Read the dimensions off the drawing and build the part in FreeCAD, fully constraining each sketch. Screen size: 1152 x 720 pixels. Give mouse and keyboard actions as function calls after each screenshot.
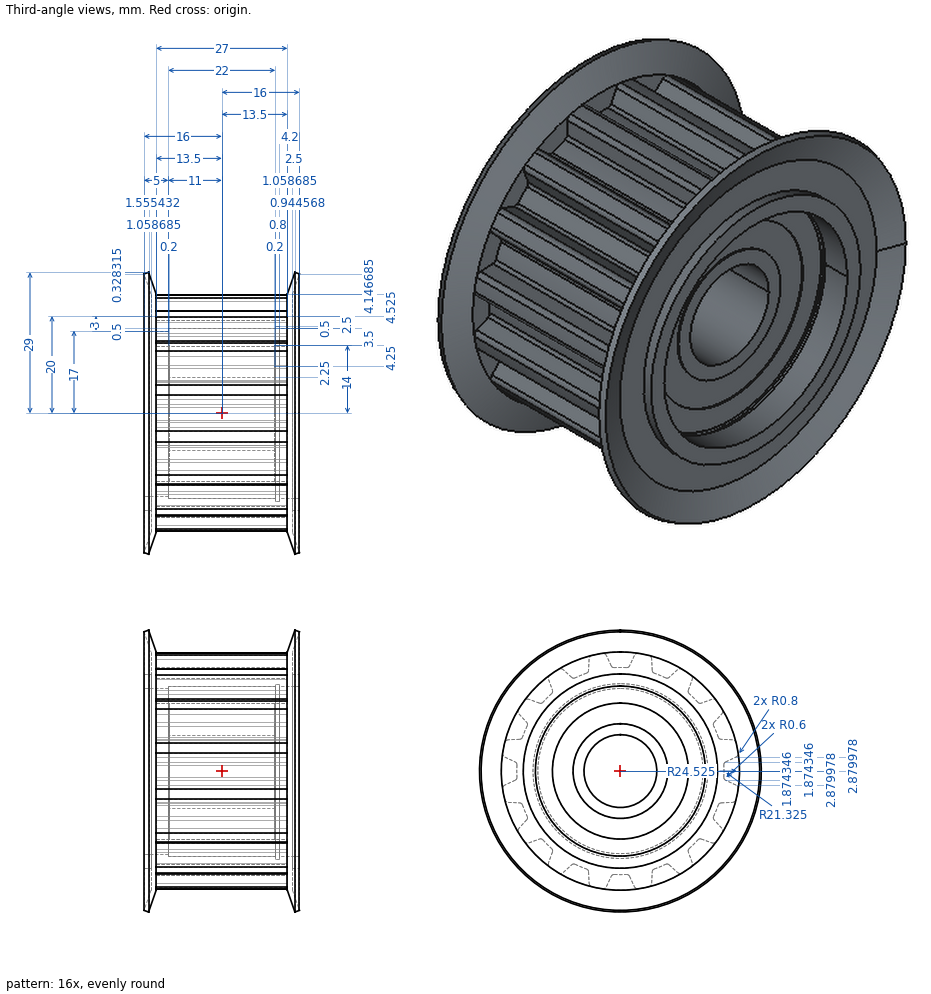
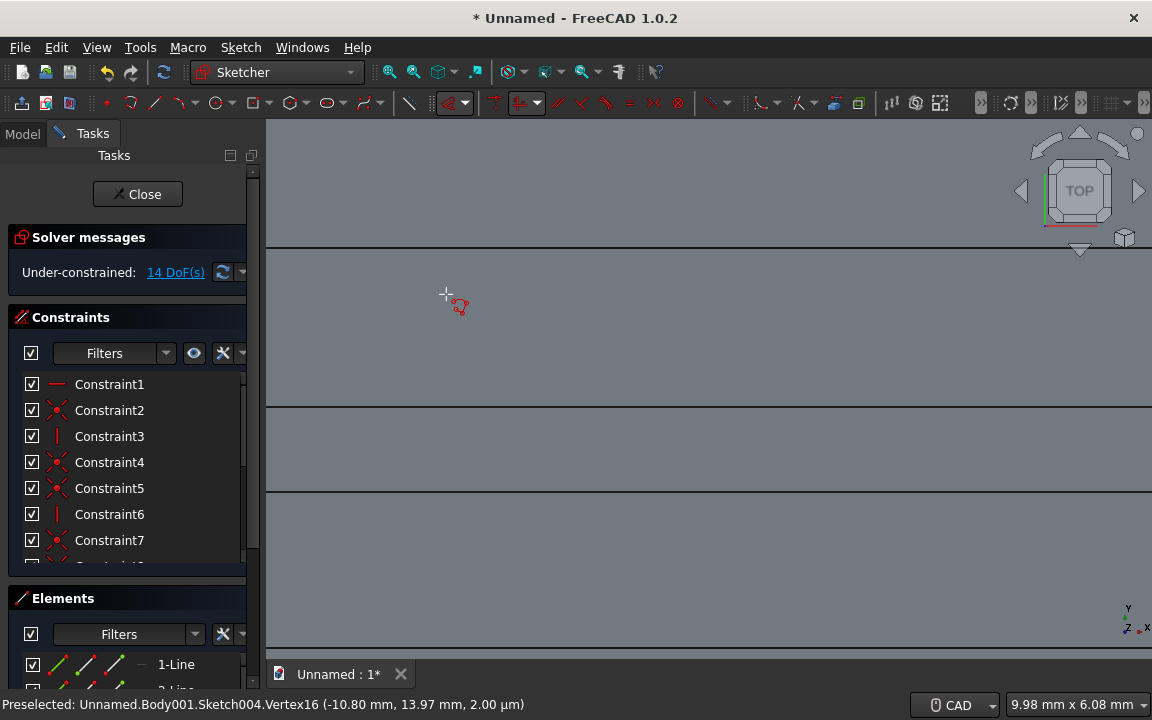
scroll(447, 295, down, 8)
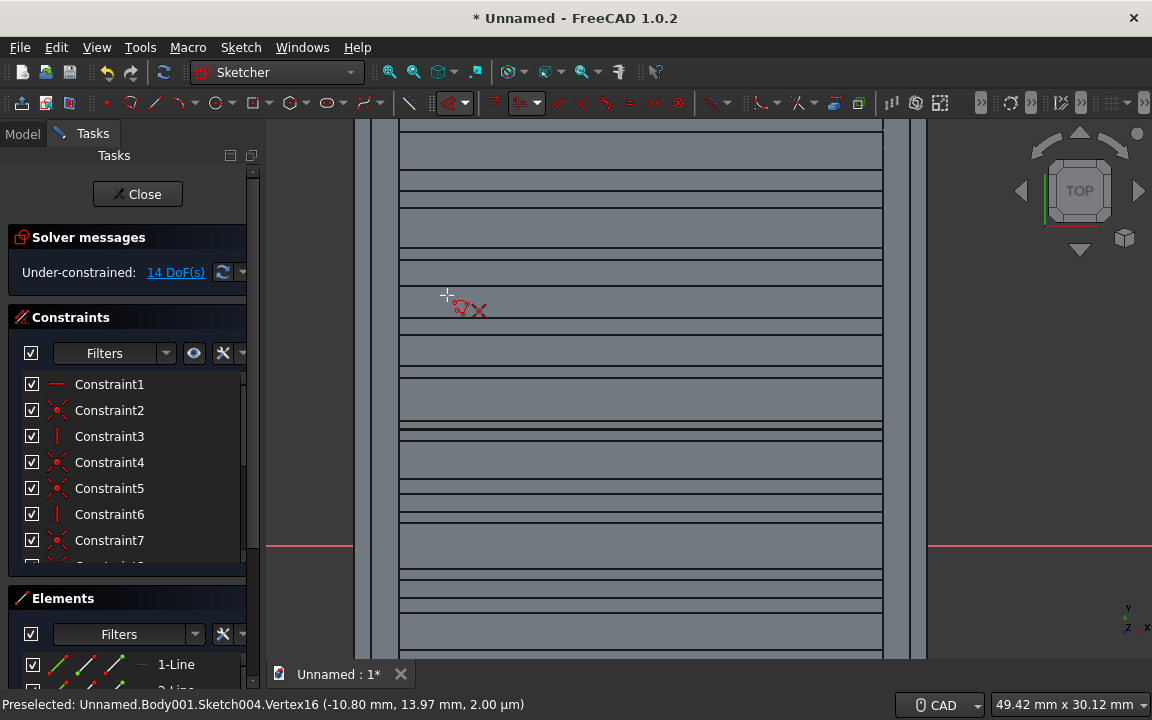
click(447, 371)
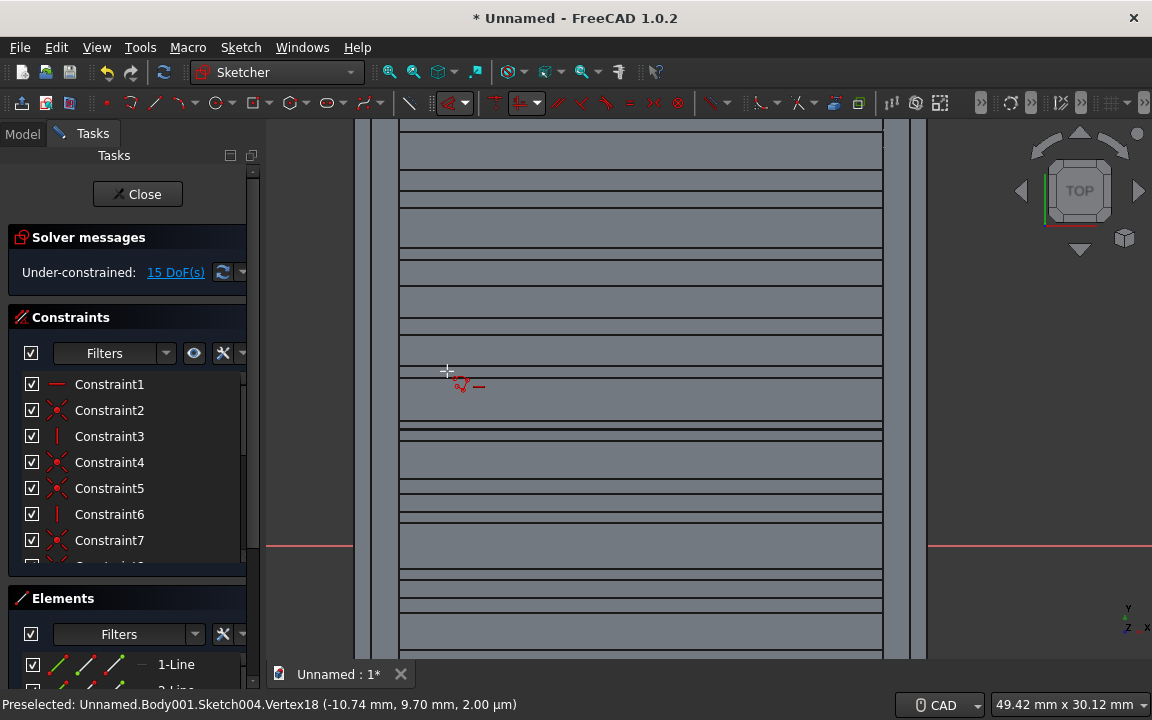
scroll(443, 371, up, 8)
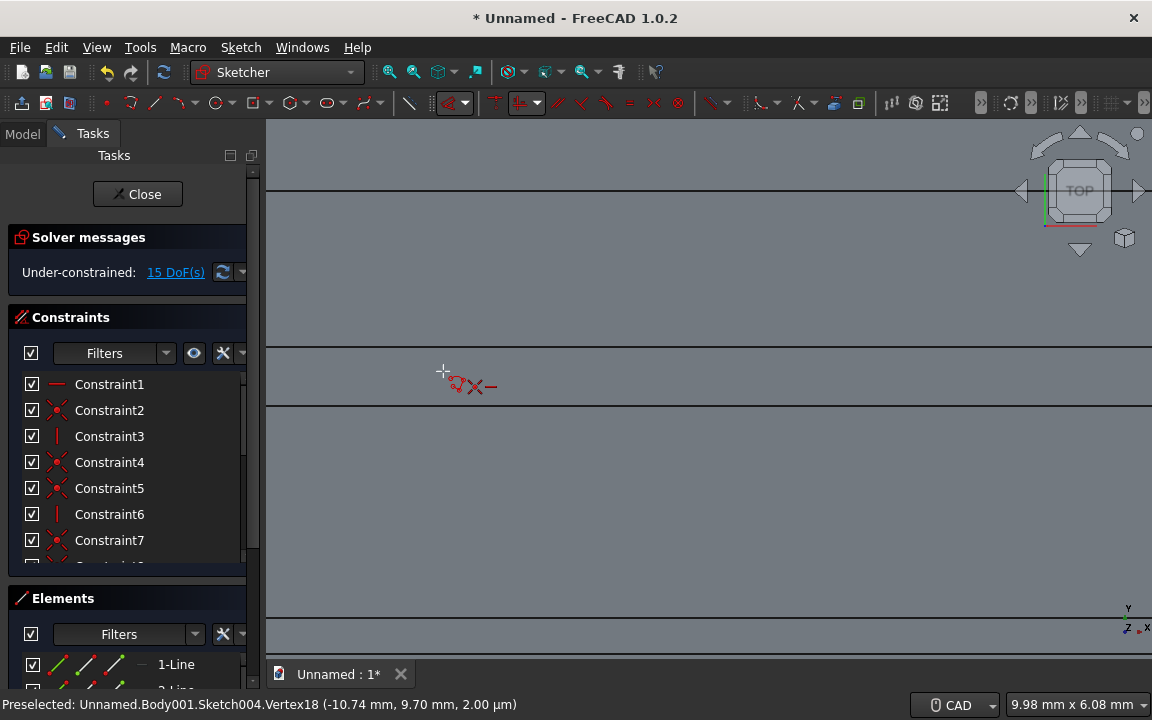
click(444, 369)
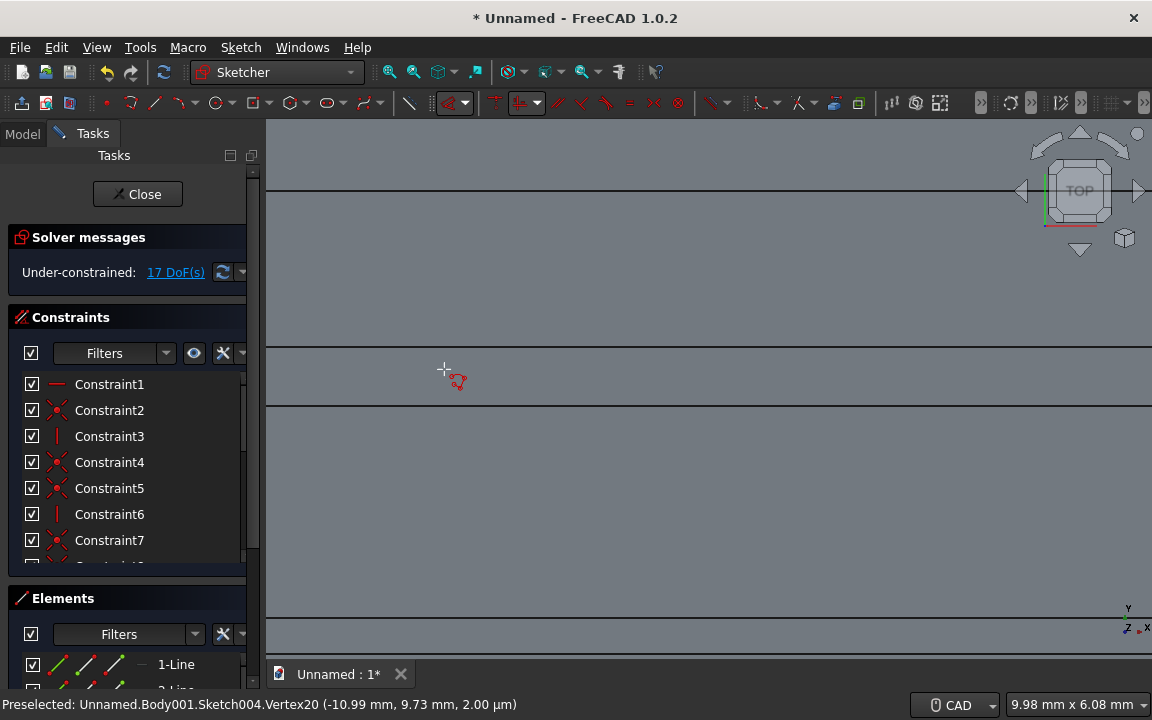
scroll(443, 371, down, 8)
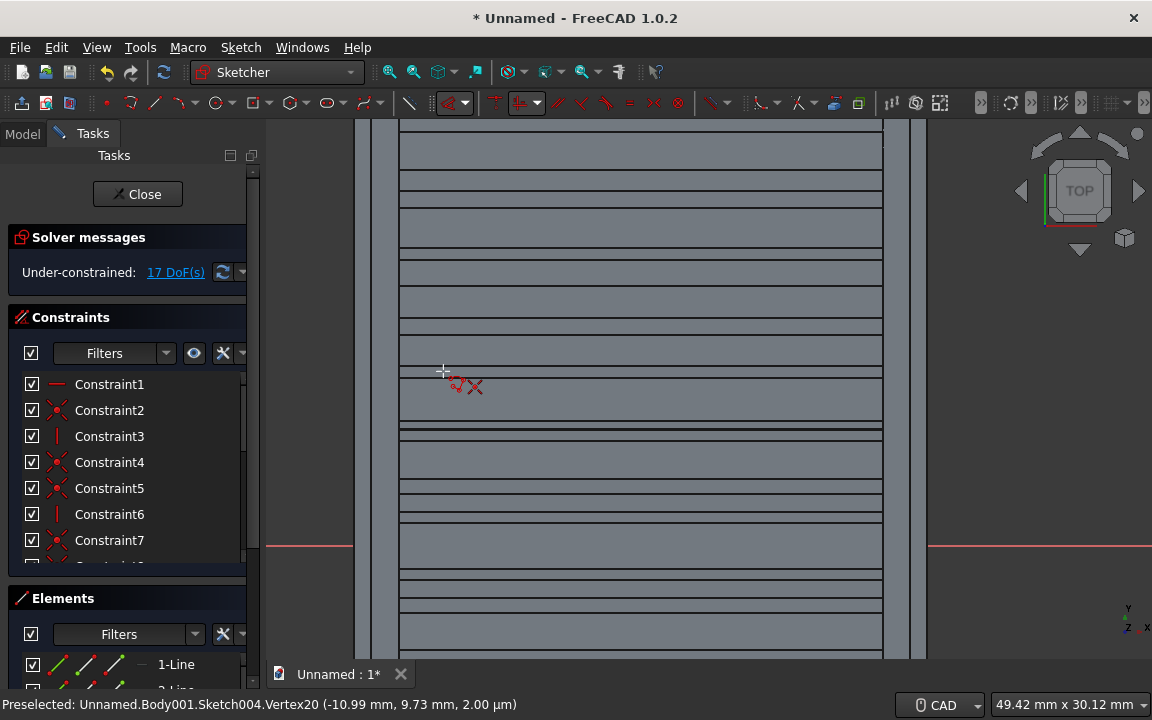
click(443, 412)
key(Escape)
key(Escape)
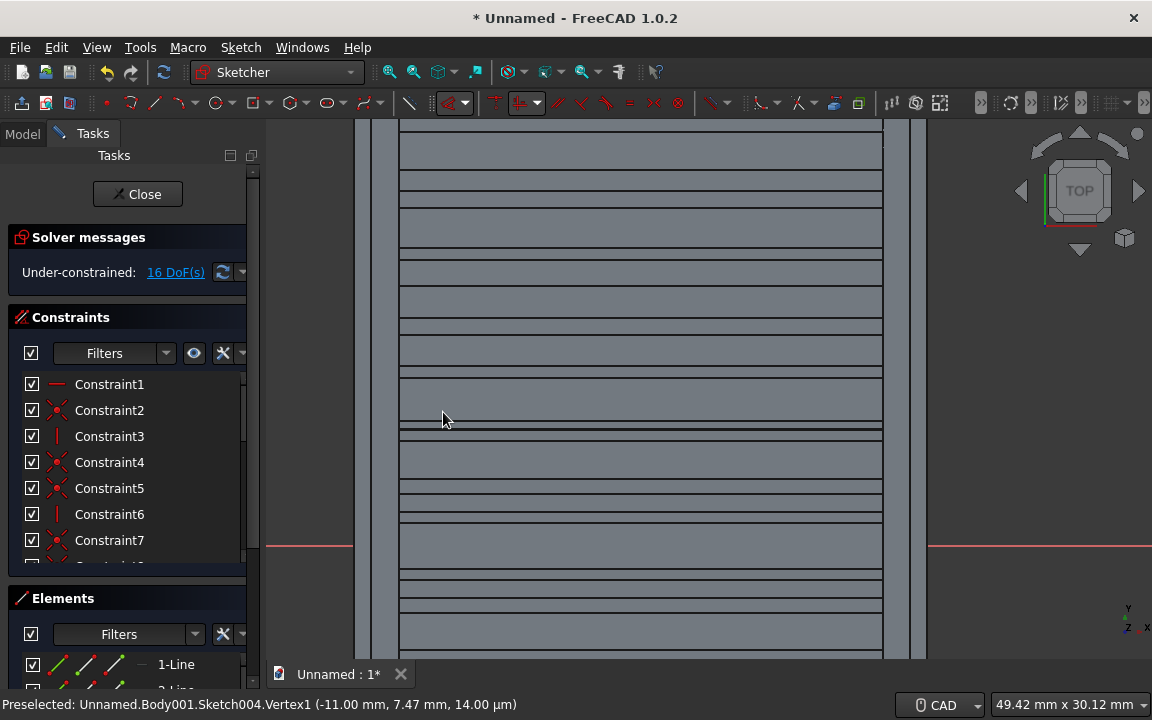
scroll(836, 372, up, 11)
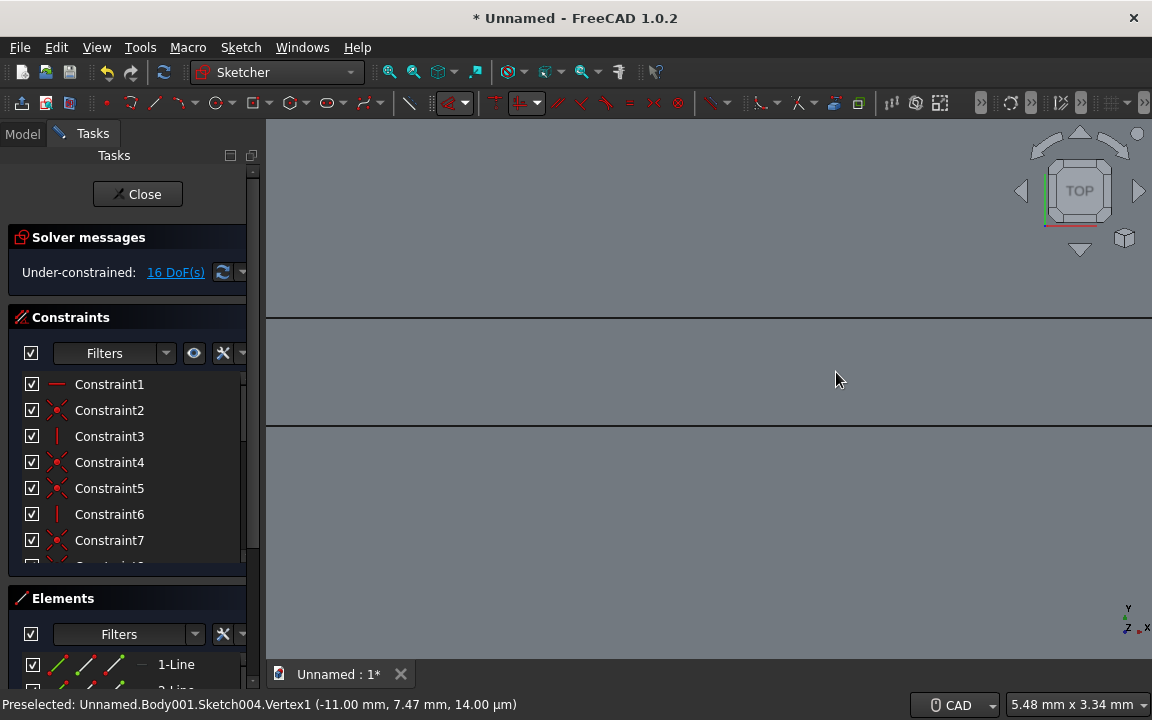
click(829, 364)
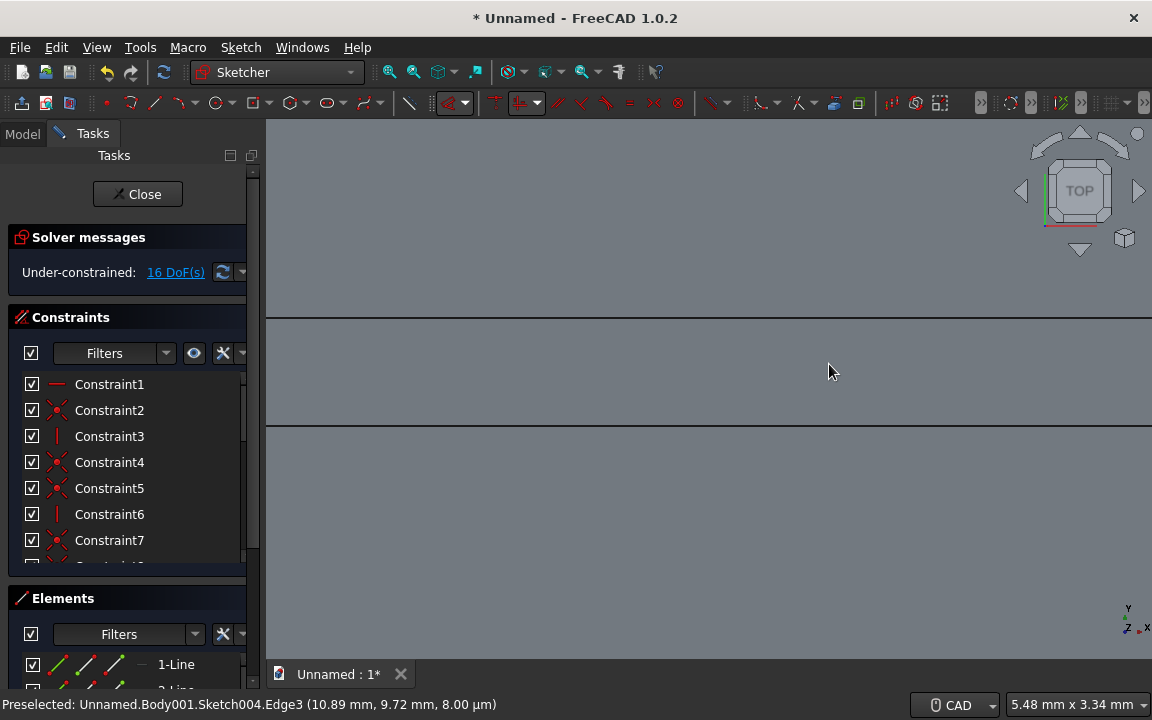
key(h)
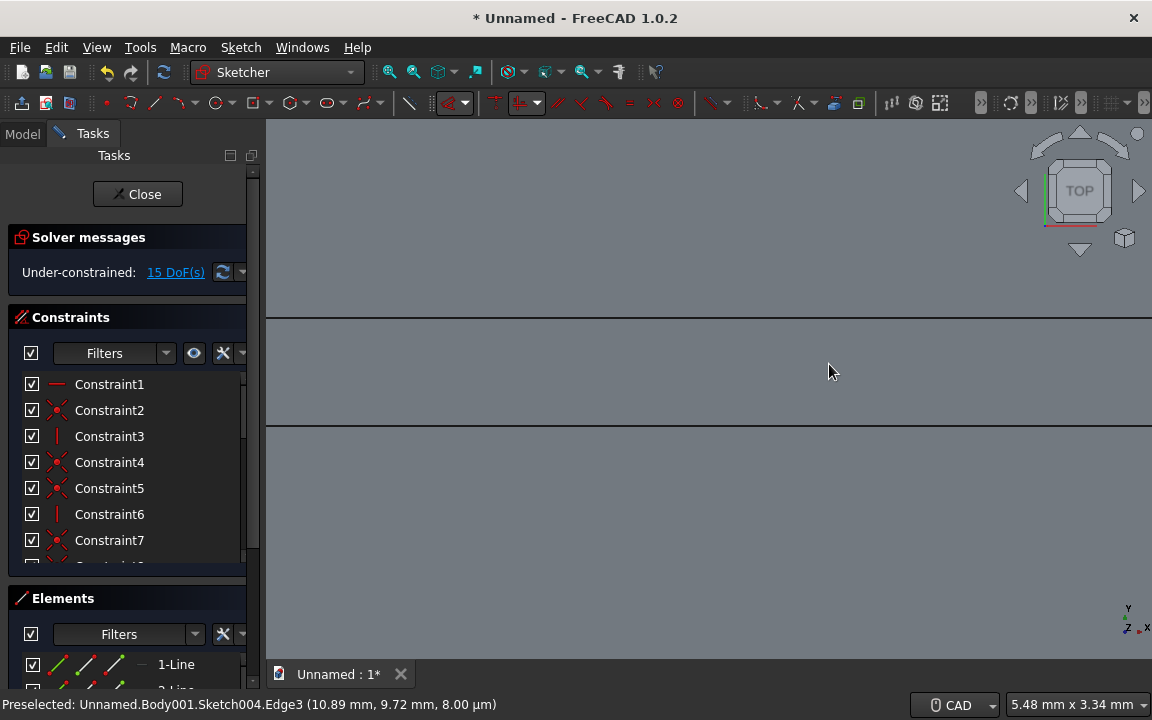
scroll(837, 372, down, 11)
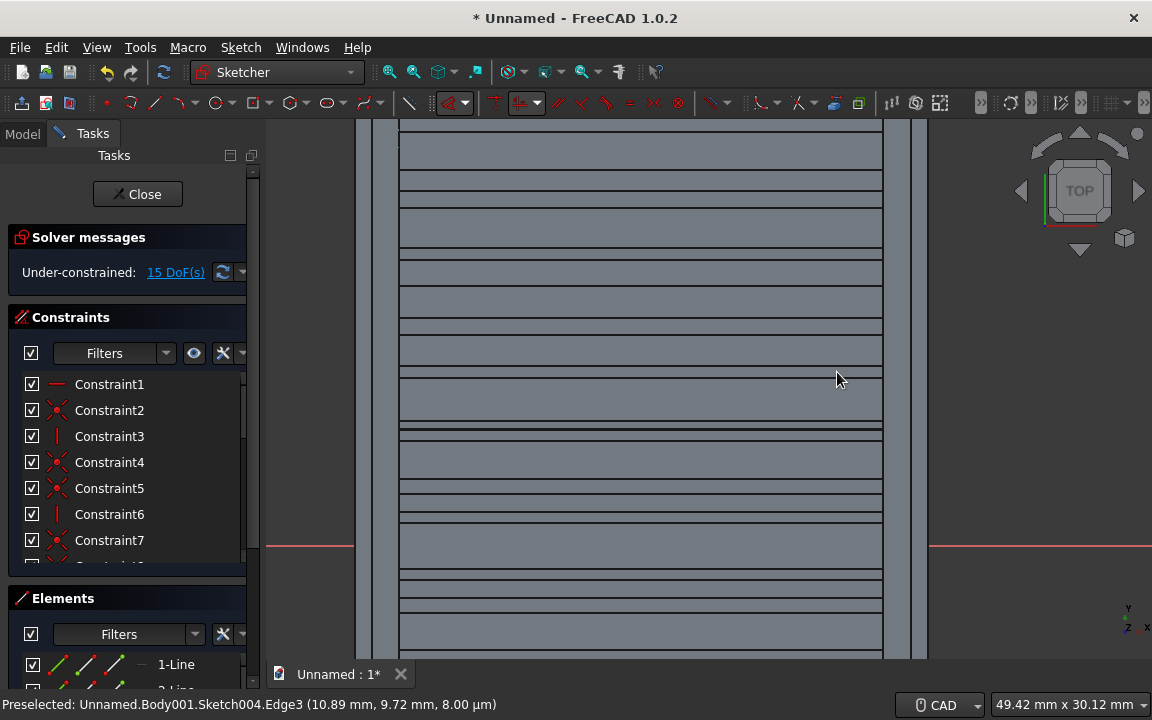
scroll(836, 296, up, 13)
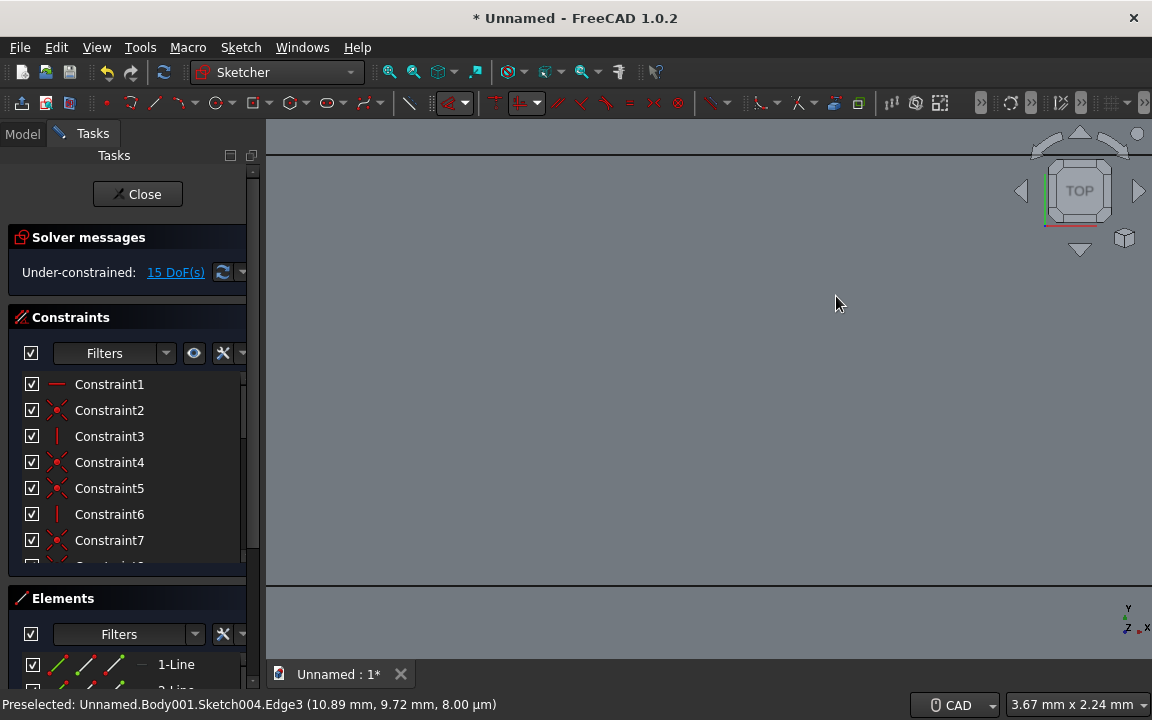
click(829, 289)